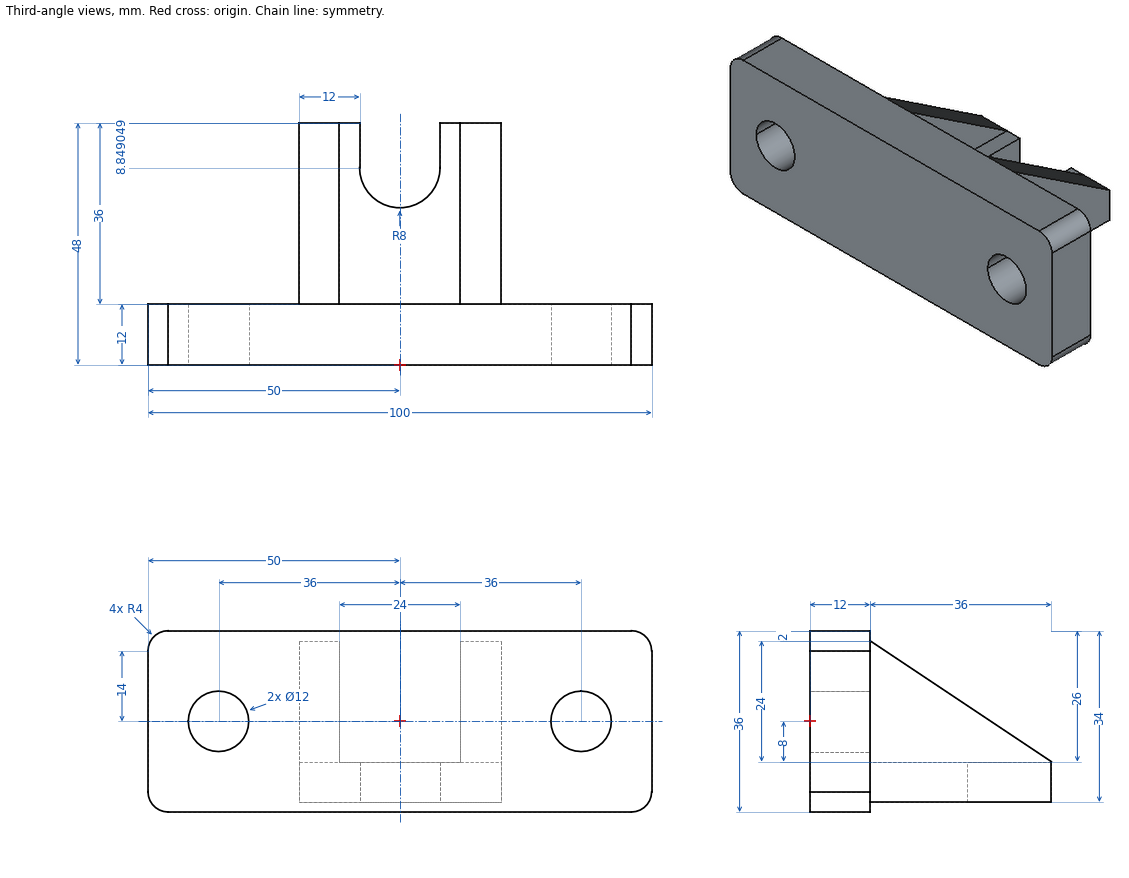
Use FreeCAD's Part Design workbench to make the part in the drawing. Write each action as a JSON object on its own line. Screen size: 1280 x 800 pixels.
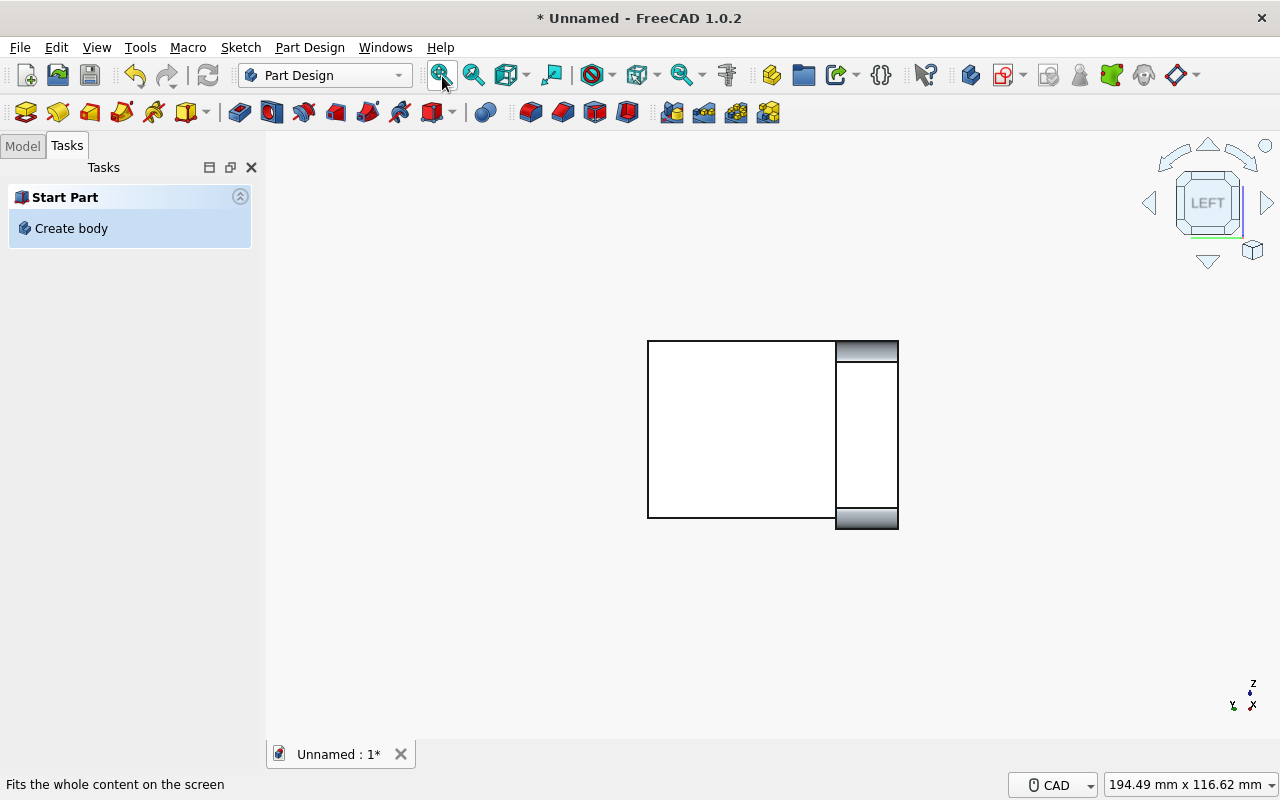
{"action": "left_click", "coordinate": [742, 429]}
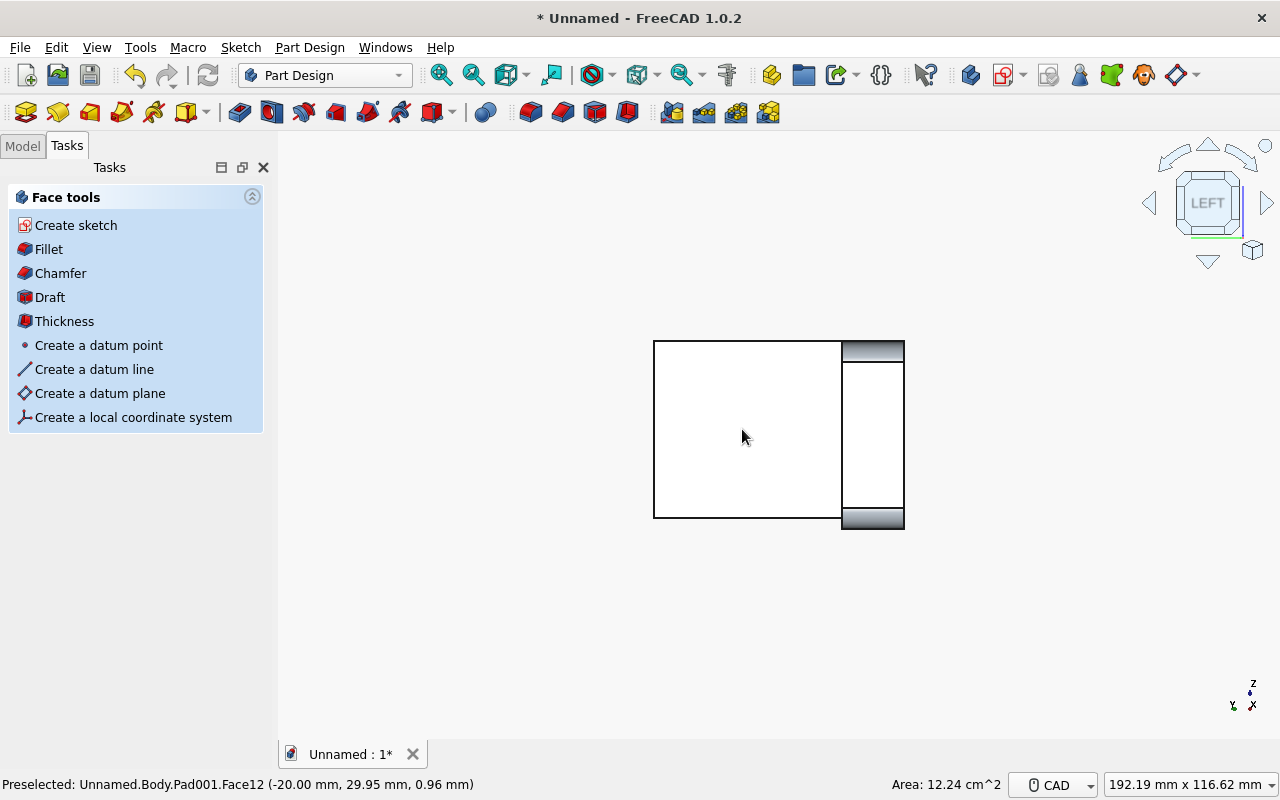
{"action": "left_click", "coordinate": [1004, 76]}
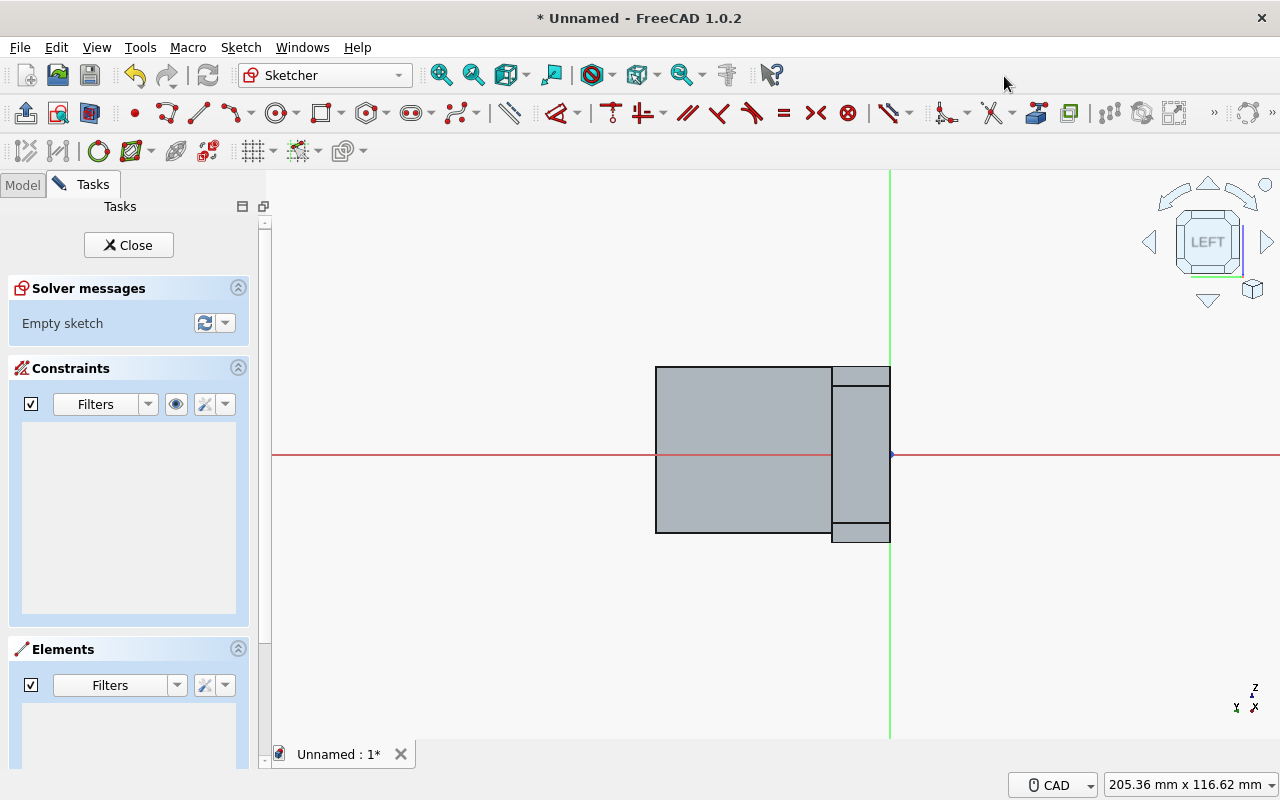
{"action": "scroll", "coordinate": [813, 416], "scroll_direction": "up", "scroll_amount": 5}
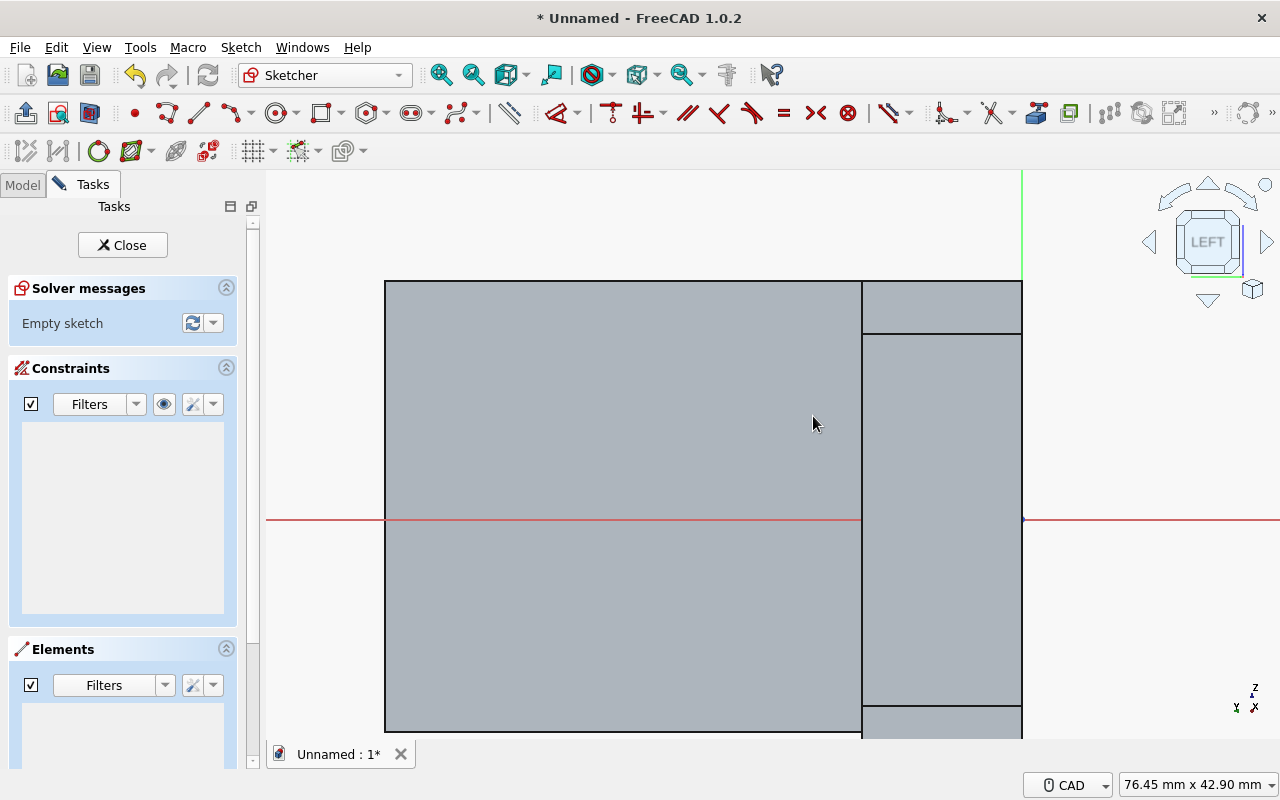
{"action": "left_click", "coordinate": [168, 114]}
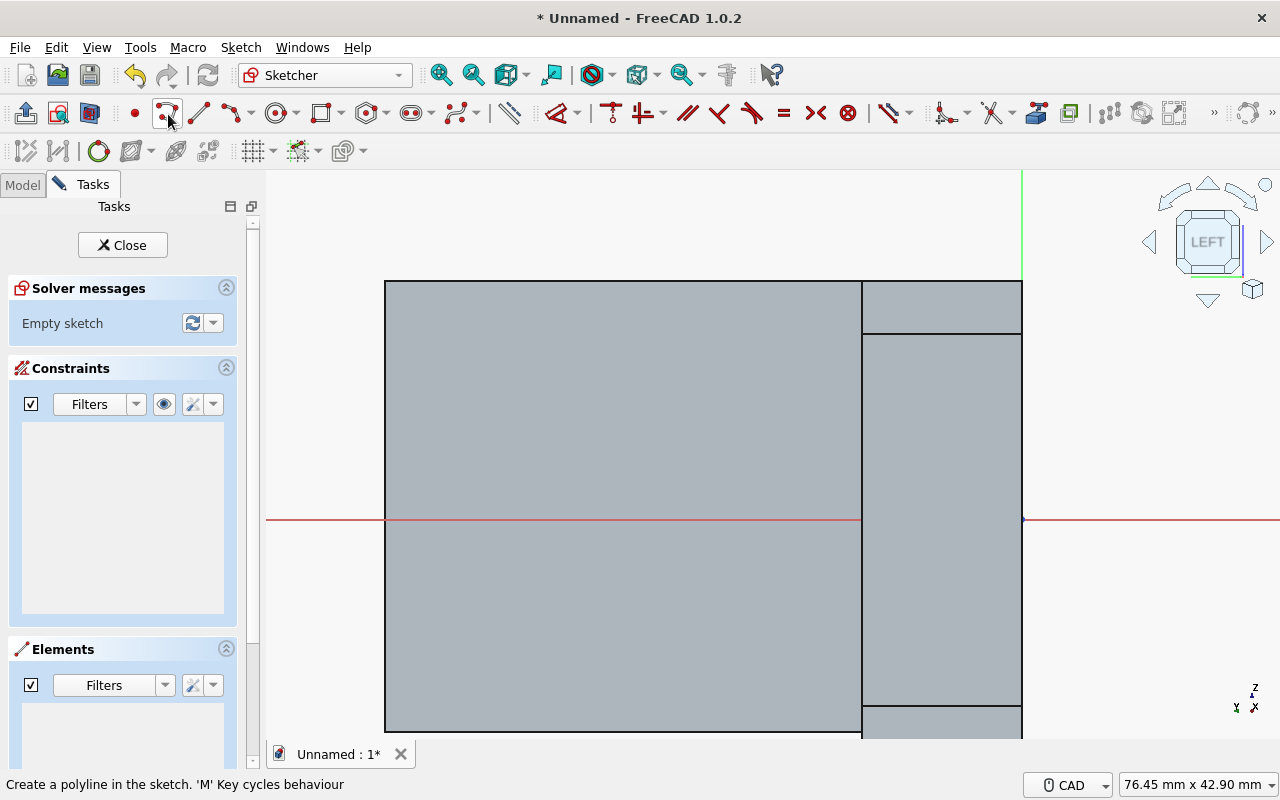
{"action": "left_click", "coordinate": [862, 308]}
{"action": "left_click", "coordinate": [862, 281]}
{"action": "left_click", "coordinate": [385, 281]}
{"action": "left_click", "coordinate": [385, 626]}
{"action": "left_click", "coordinate": [862, 309]}
{"action": "key", "text": "Escape"}
{"action": "key", "text": "Escape"}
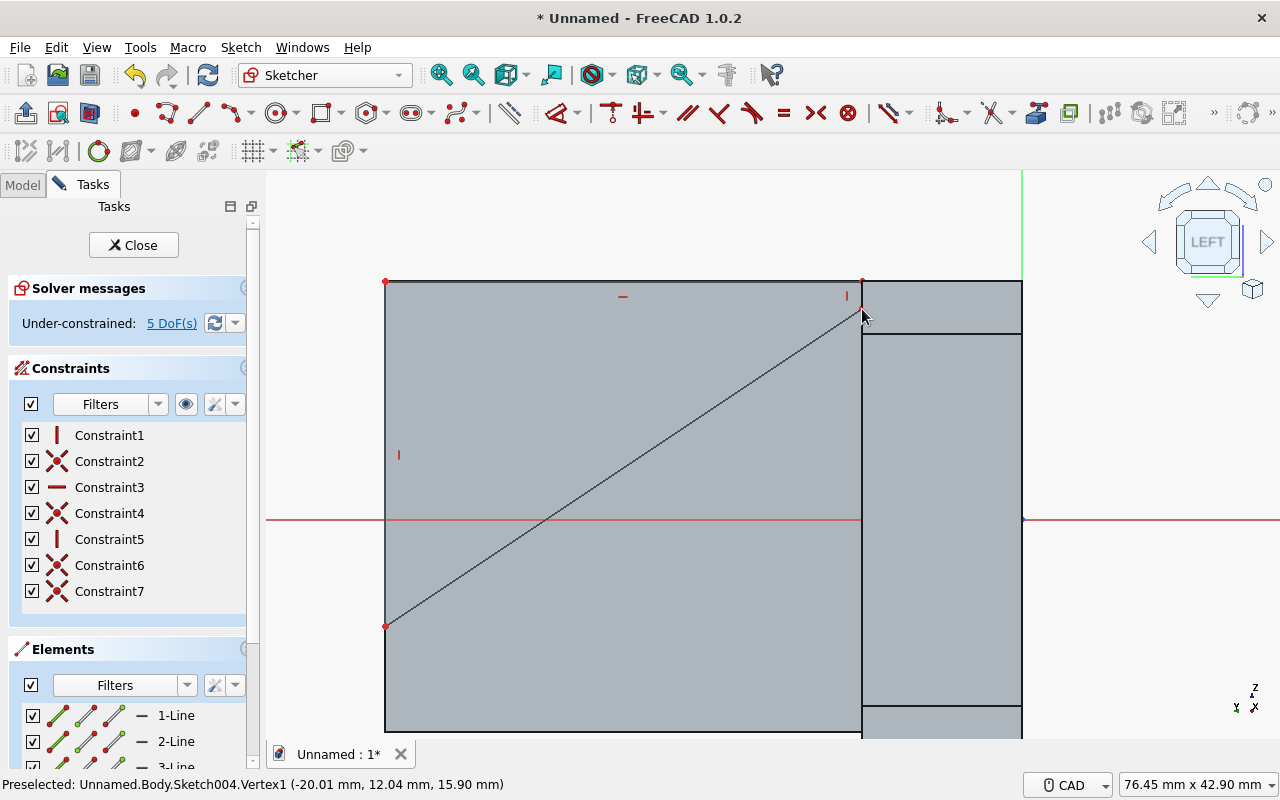
{"action": "left_click", "coordinate": [556, 114]}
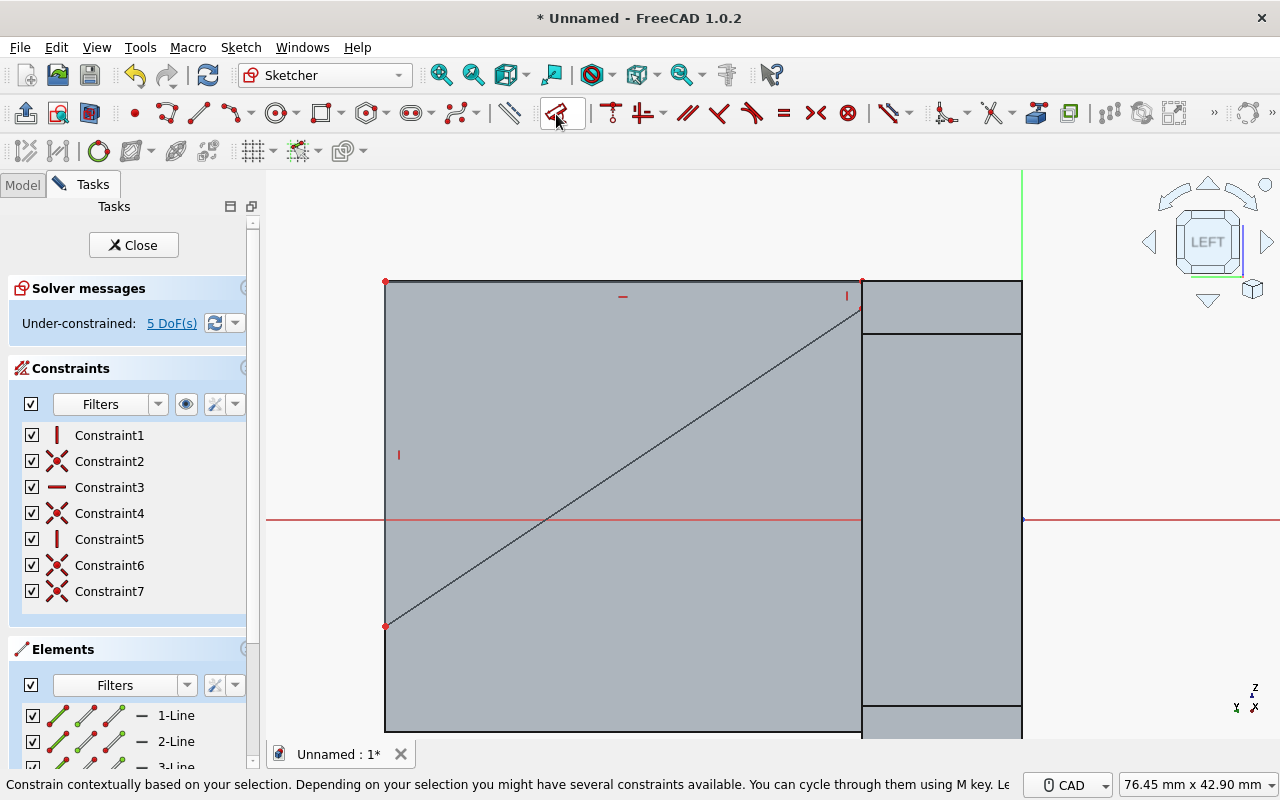
{"action": "scroll", "coordinate": [862, 298], "scroll_direction": "up", "scroll_amount": 3}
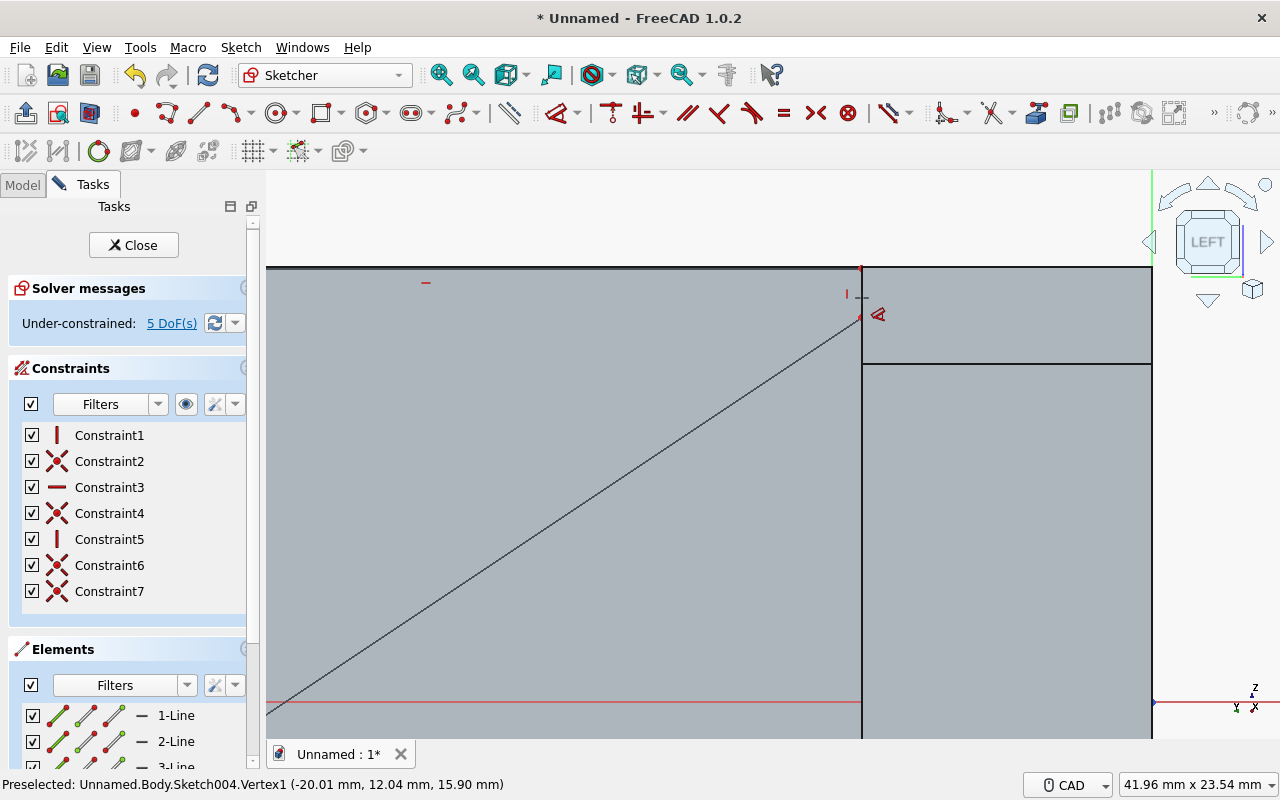
{"action": "left_click", "coordinate": [862, 298]}
{"action": "left_click", "coordinate": [896, 293]}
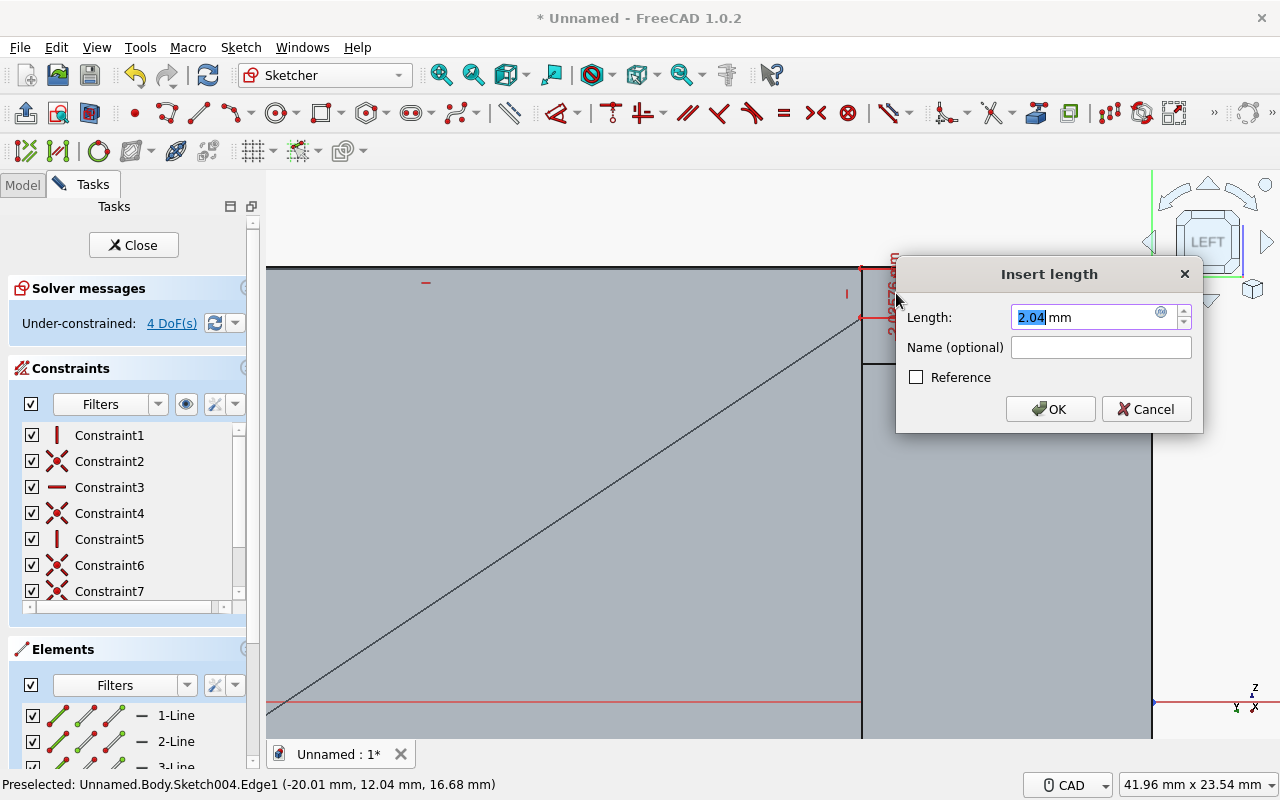
{"action": "type", "text": "2"}
{"action": "key", "text": "Return"}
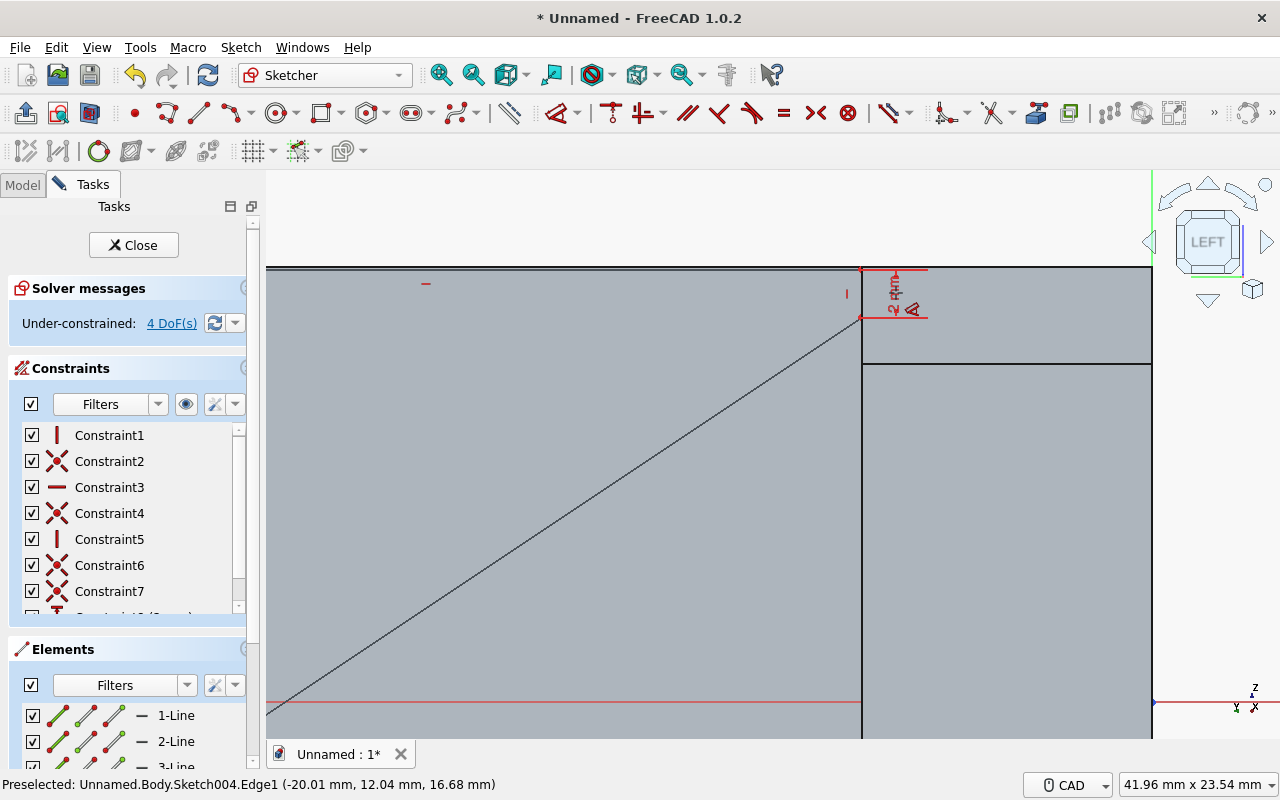
{"action": "left_click", "coordinate": [601, 270]}
{"action": "left_click", "coordinate": [578, 236]}